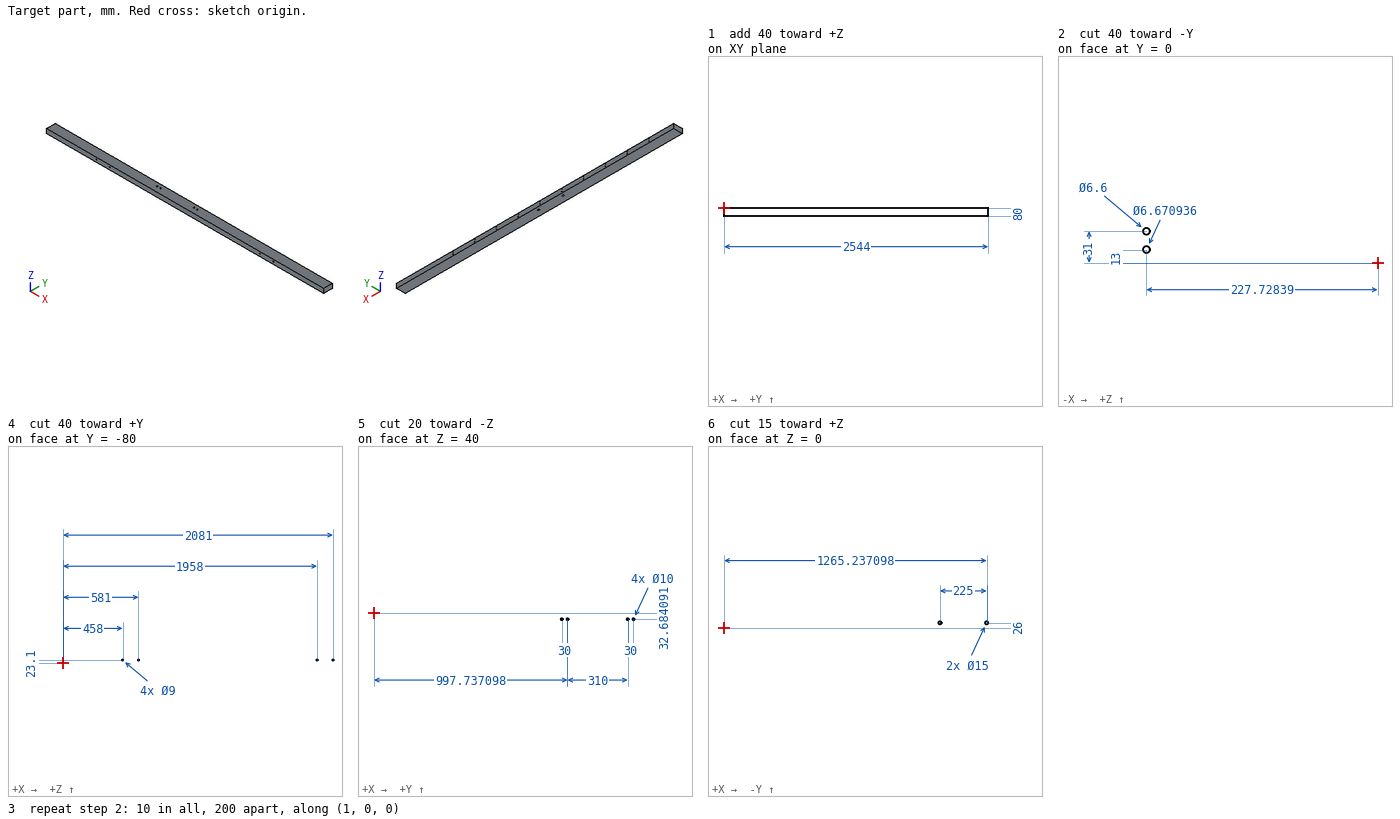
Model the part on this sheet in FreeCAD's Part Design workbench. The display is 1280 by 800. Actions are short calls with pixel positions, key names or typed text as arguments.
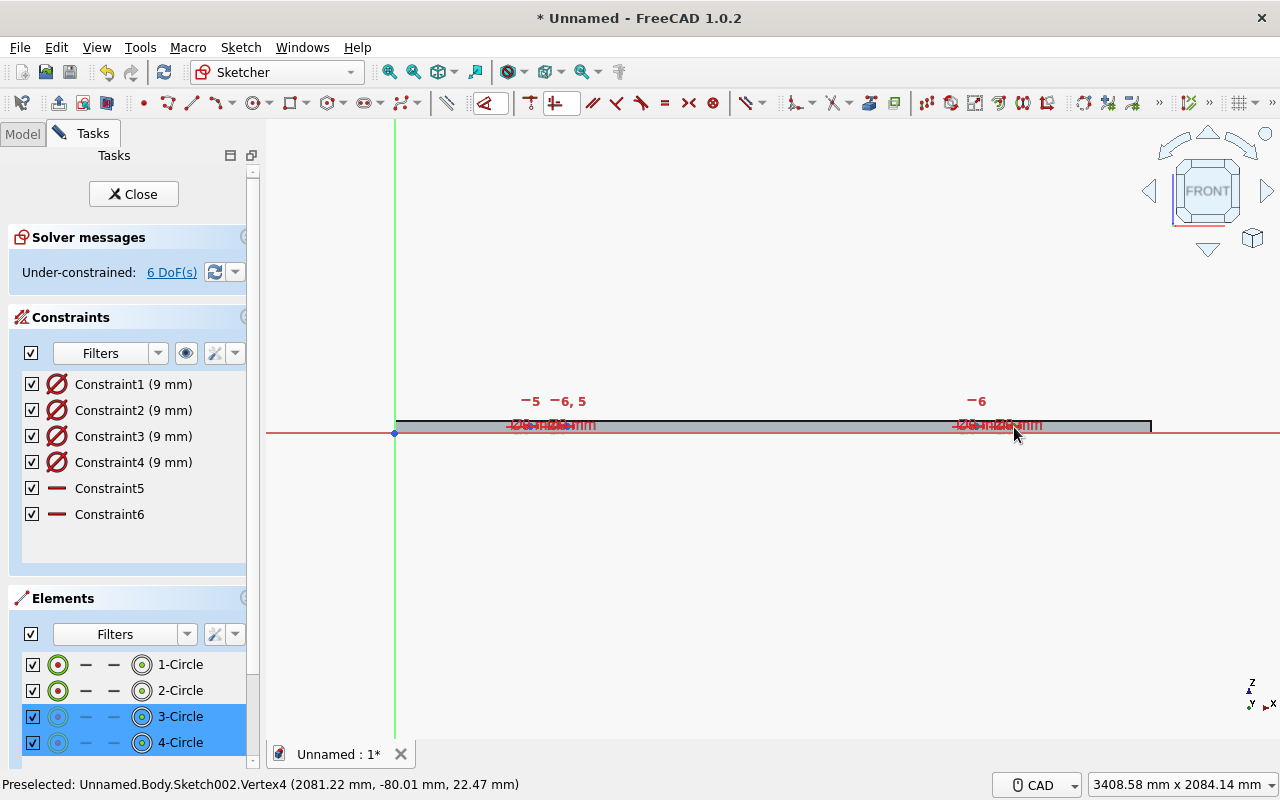
key(h)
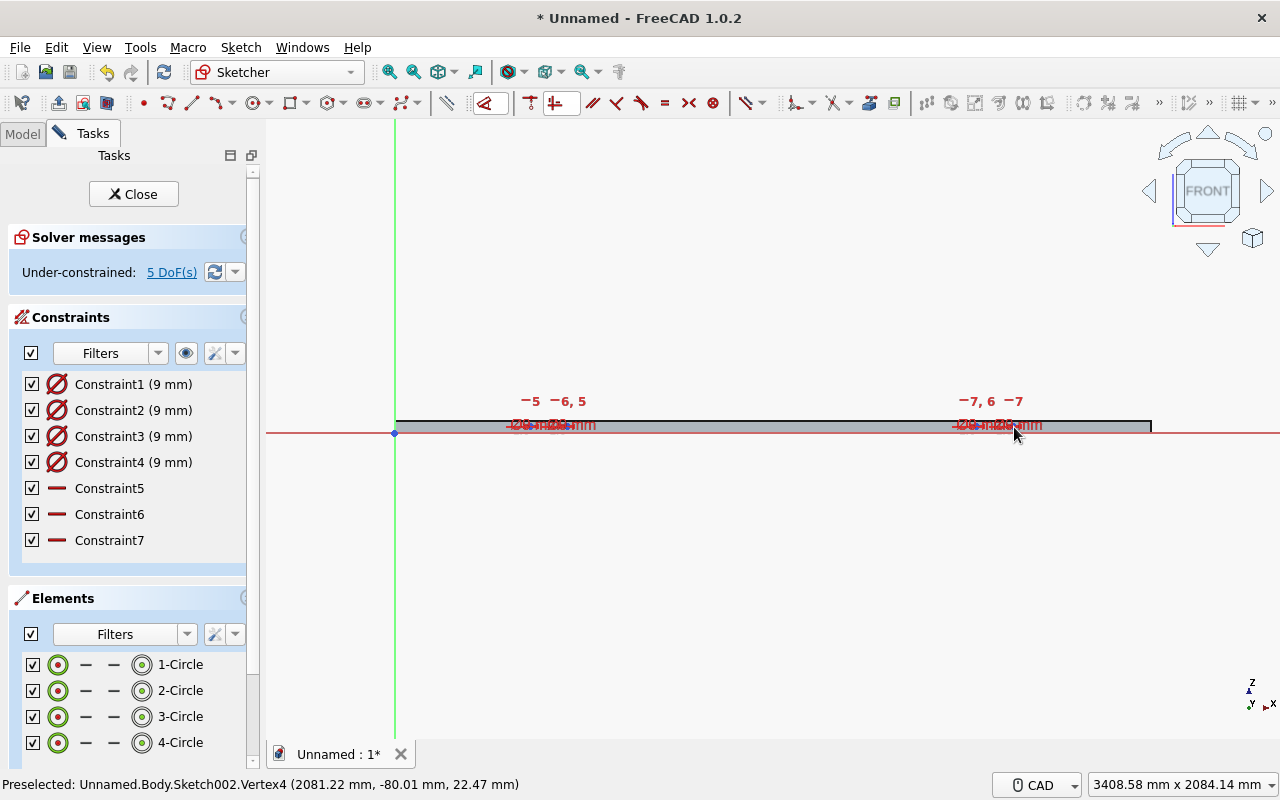
key(d)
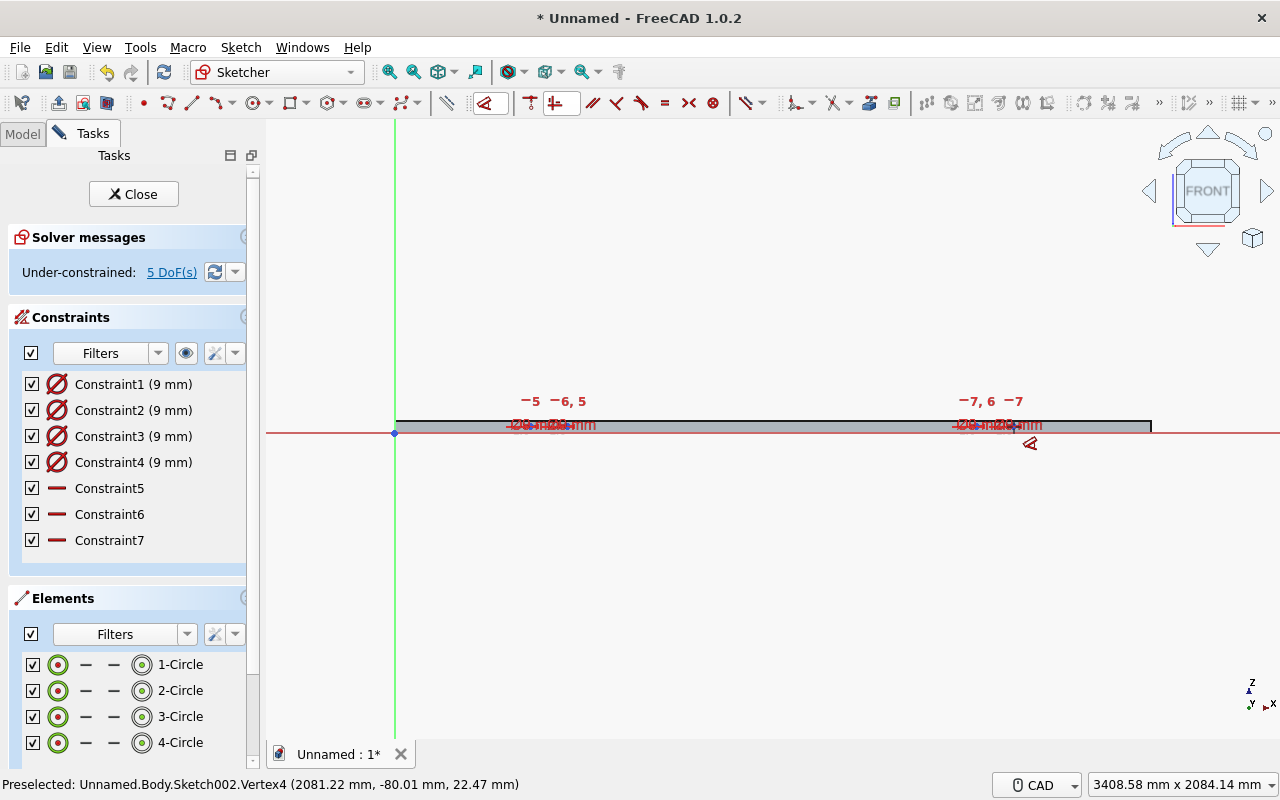
click(531, 427)
click(463, 467)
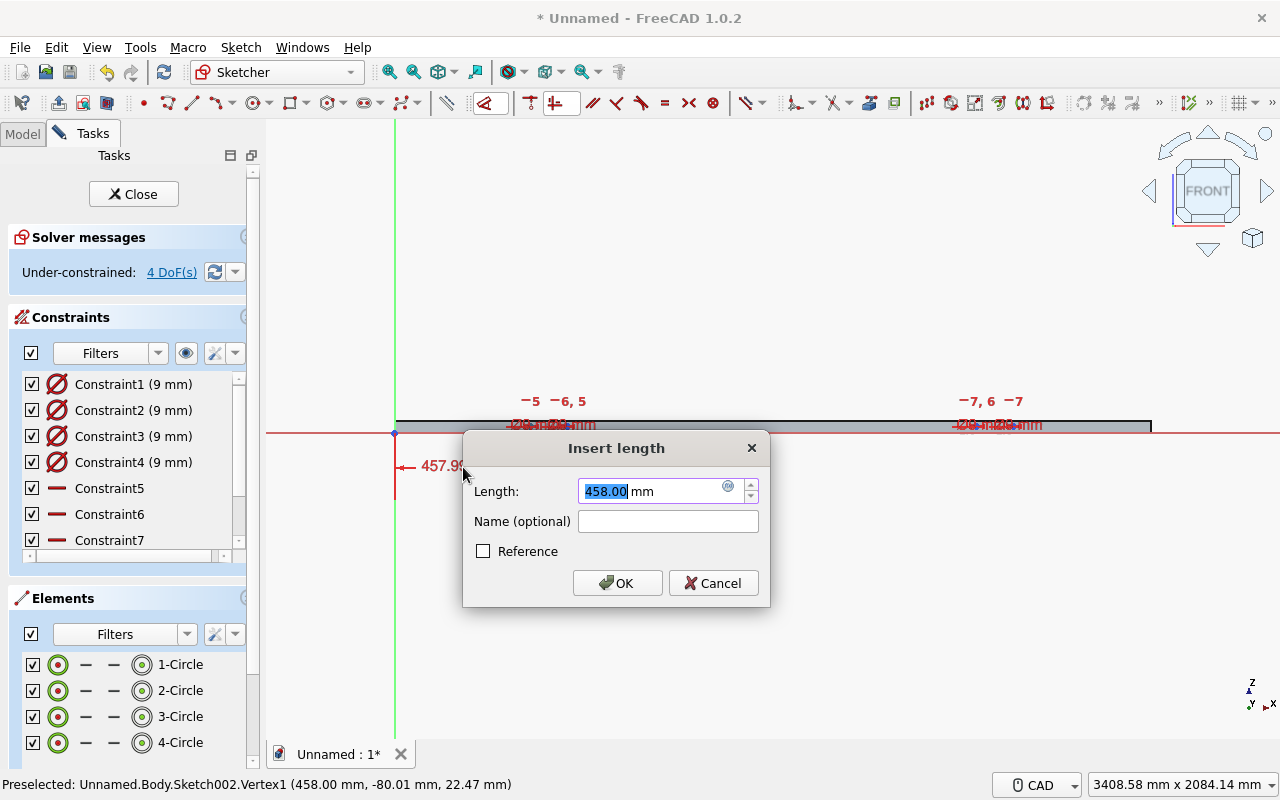
text(458)
key(Return)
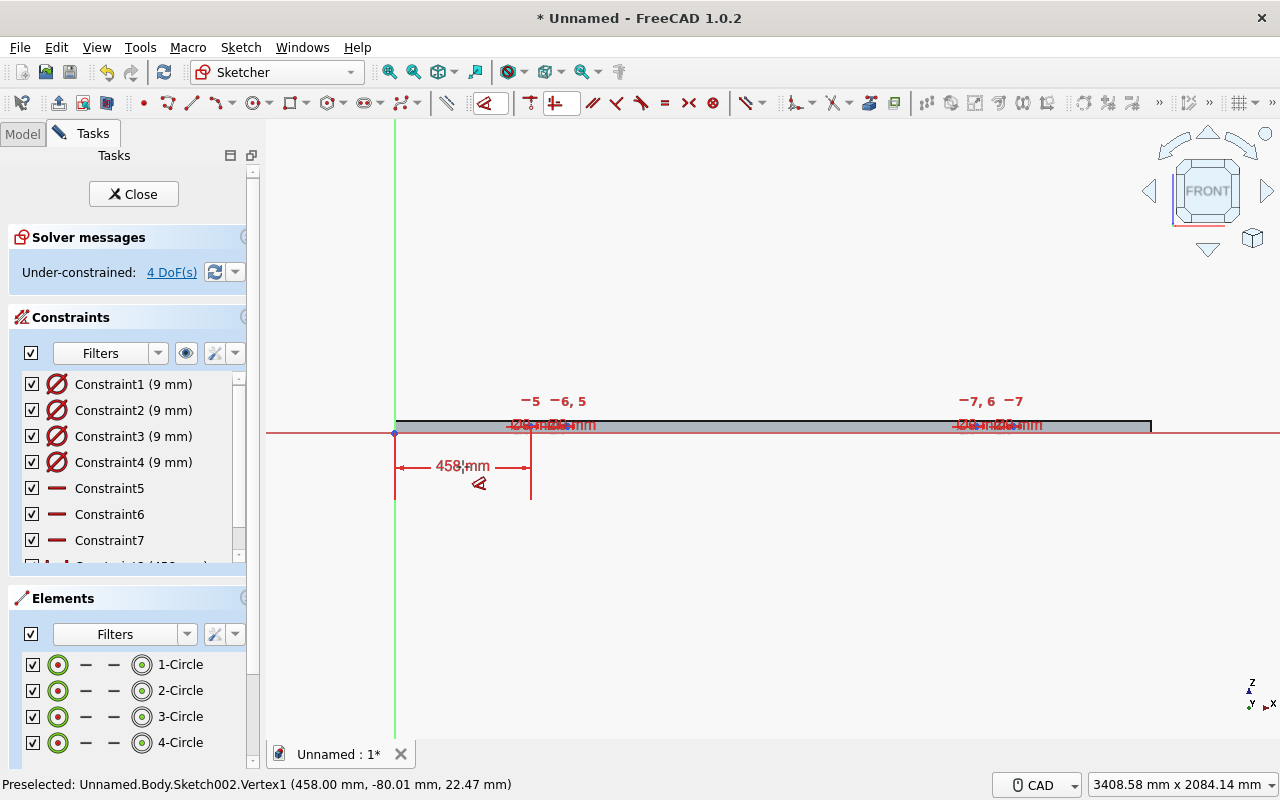
click(567, 427)
click(541, 467)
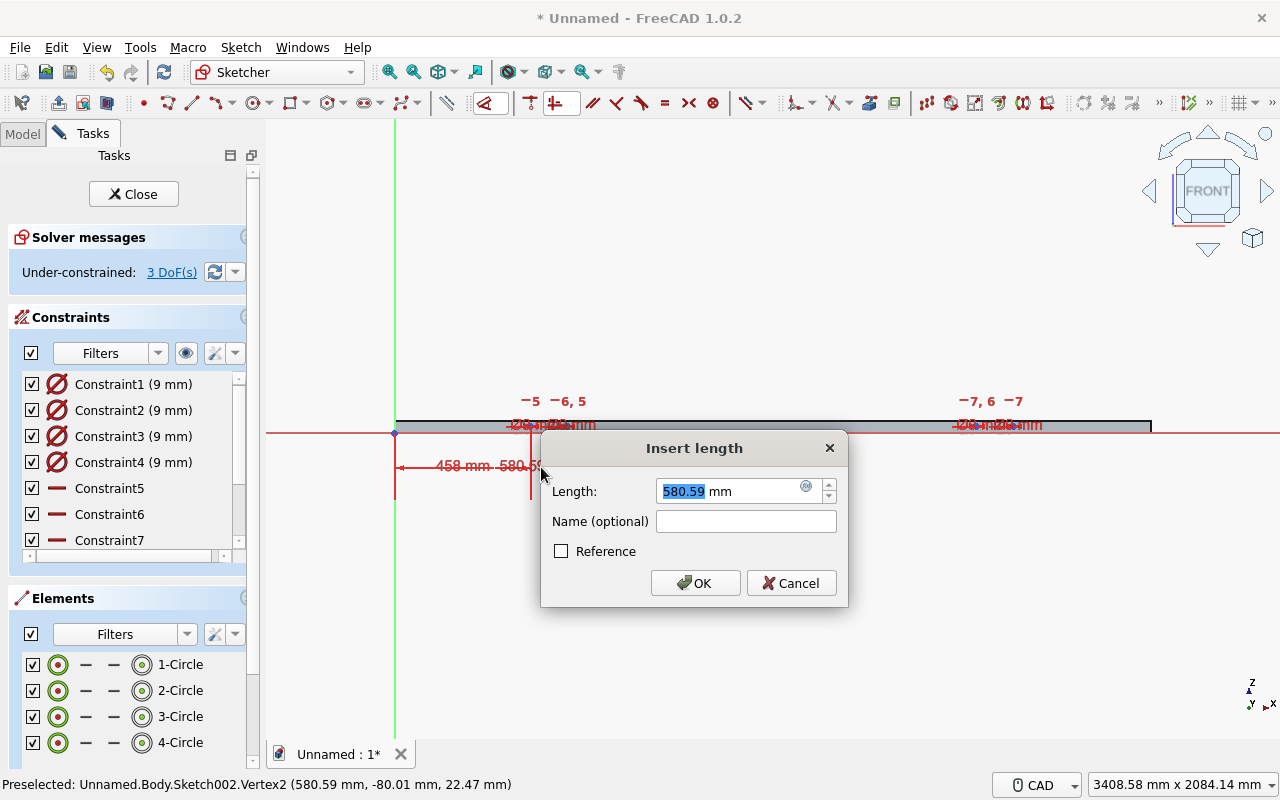
text(581)
key(Return)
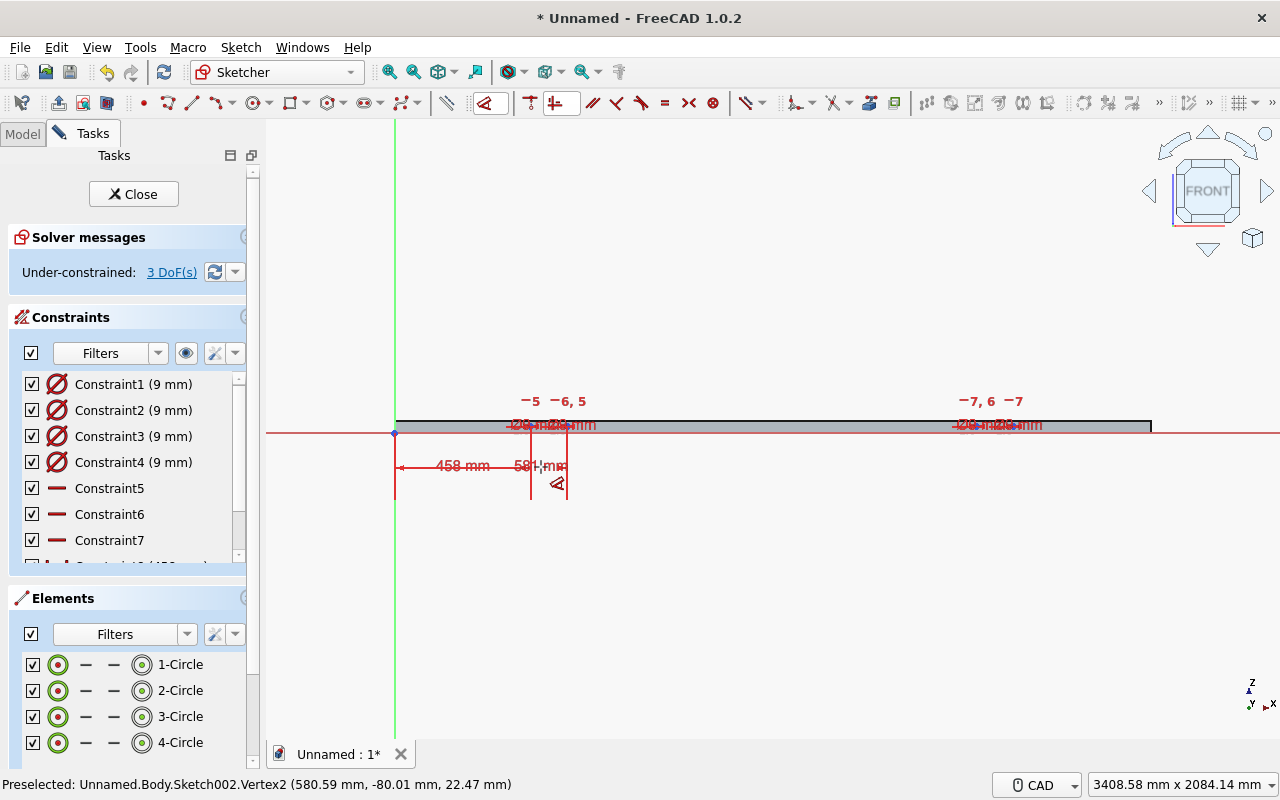
scroll(531, 427, up, 9)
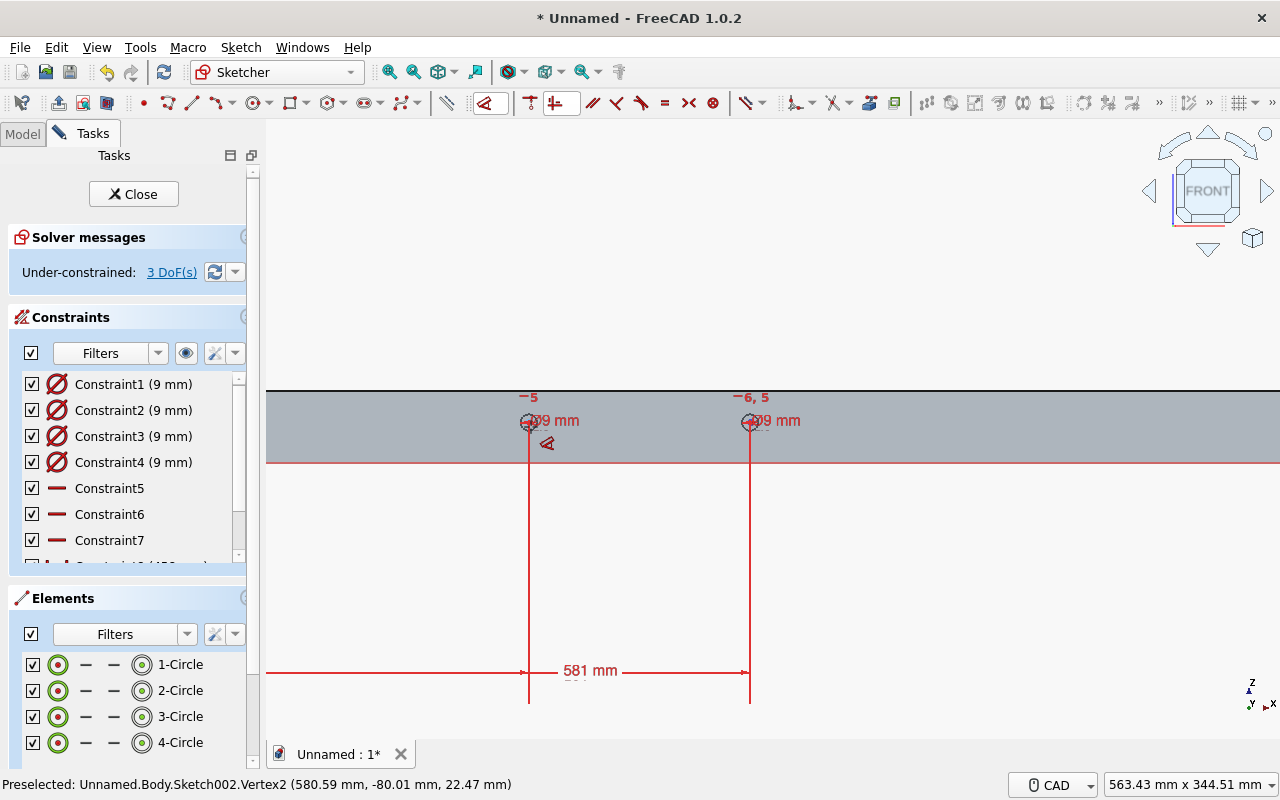
click(529, 423)
click(563, 443)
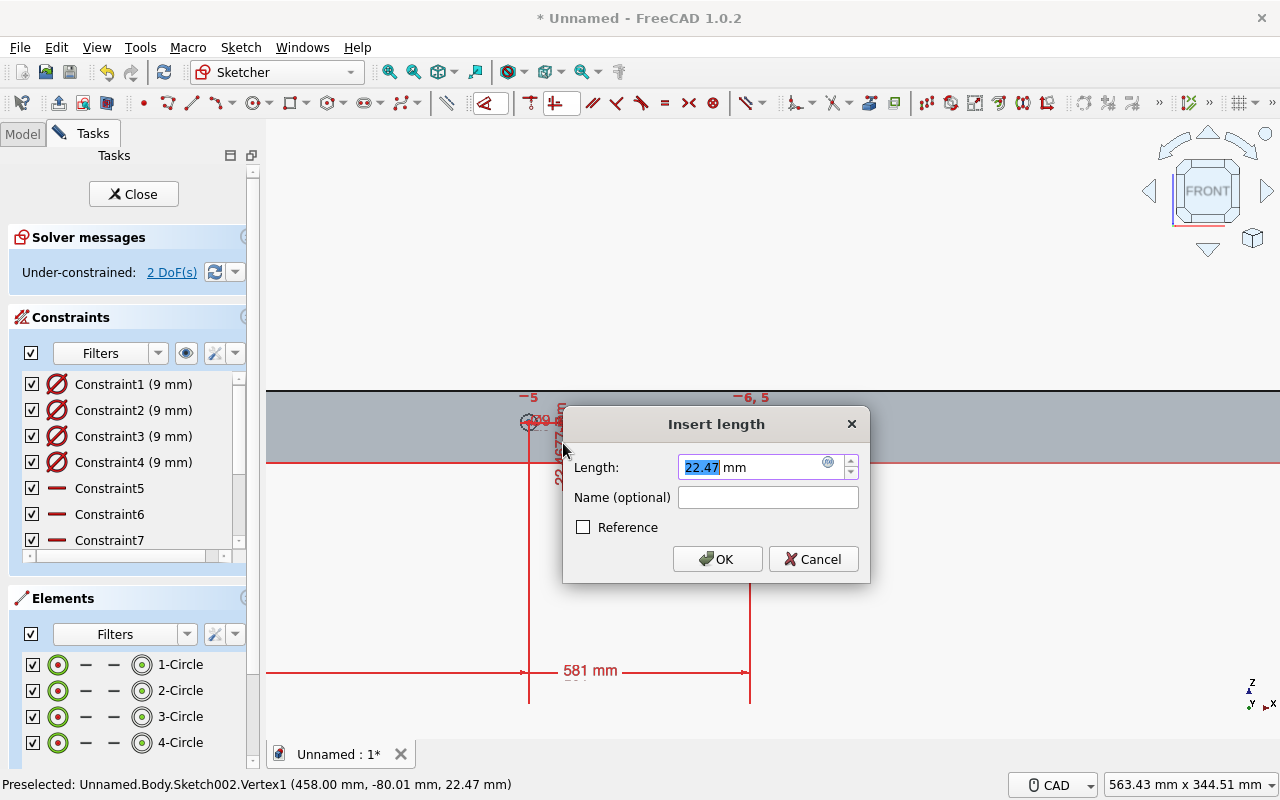
text(23.1)
key(Return)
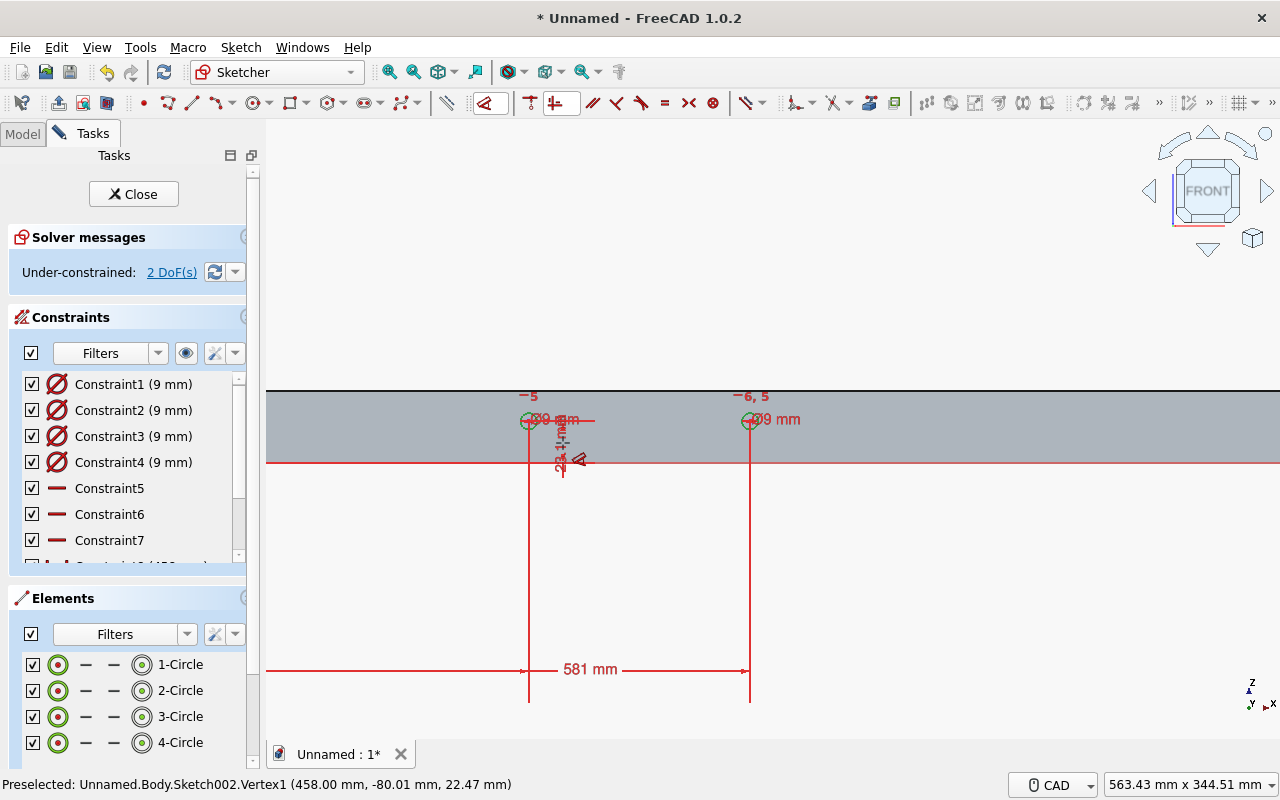
scroll(531, 427, down, 9)